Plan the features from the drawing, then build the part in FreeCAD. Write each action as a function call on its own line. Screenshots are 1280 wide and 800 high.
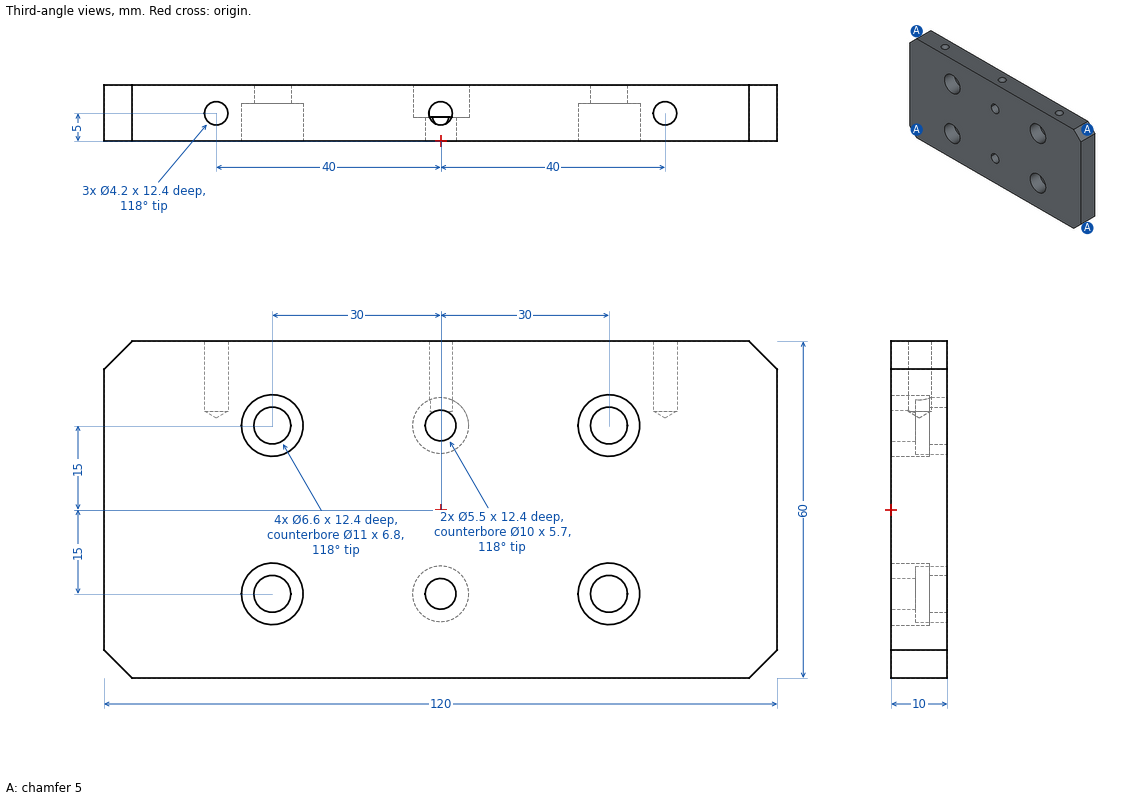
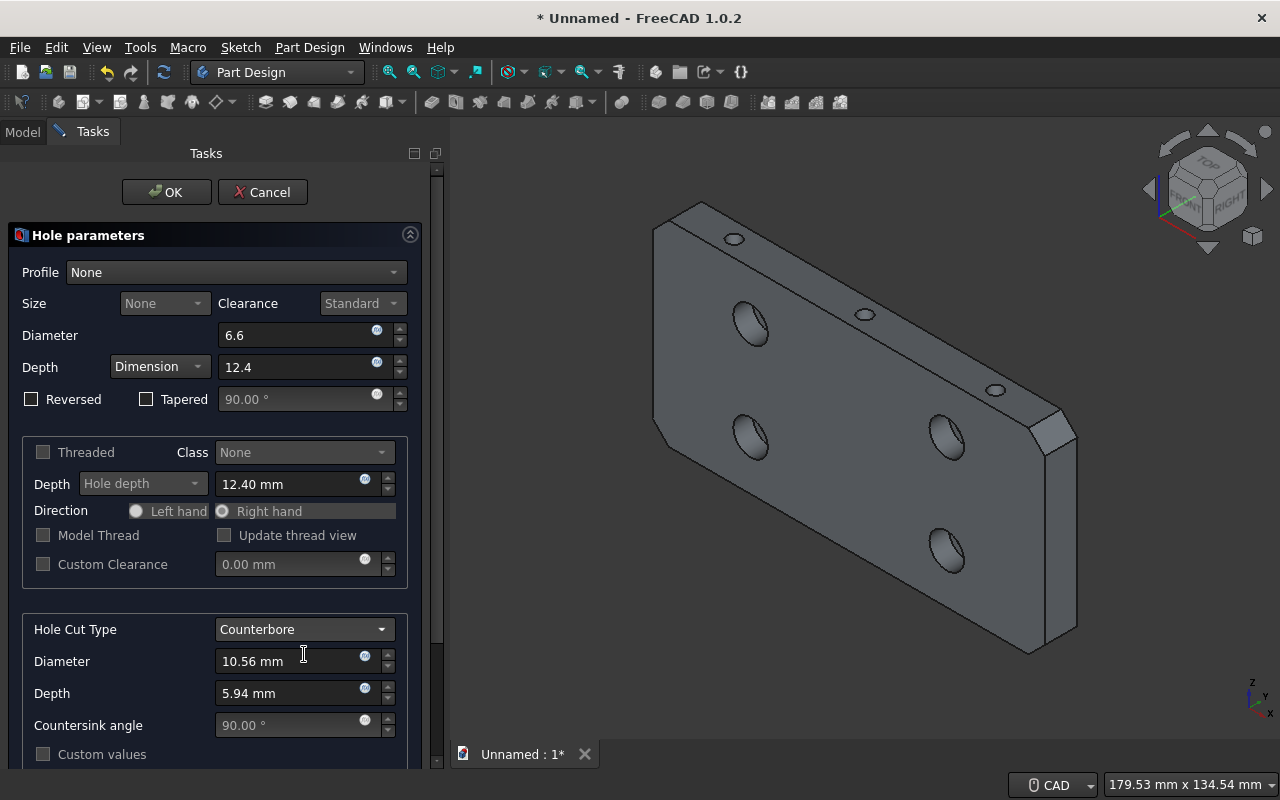
triple_click(298, 661)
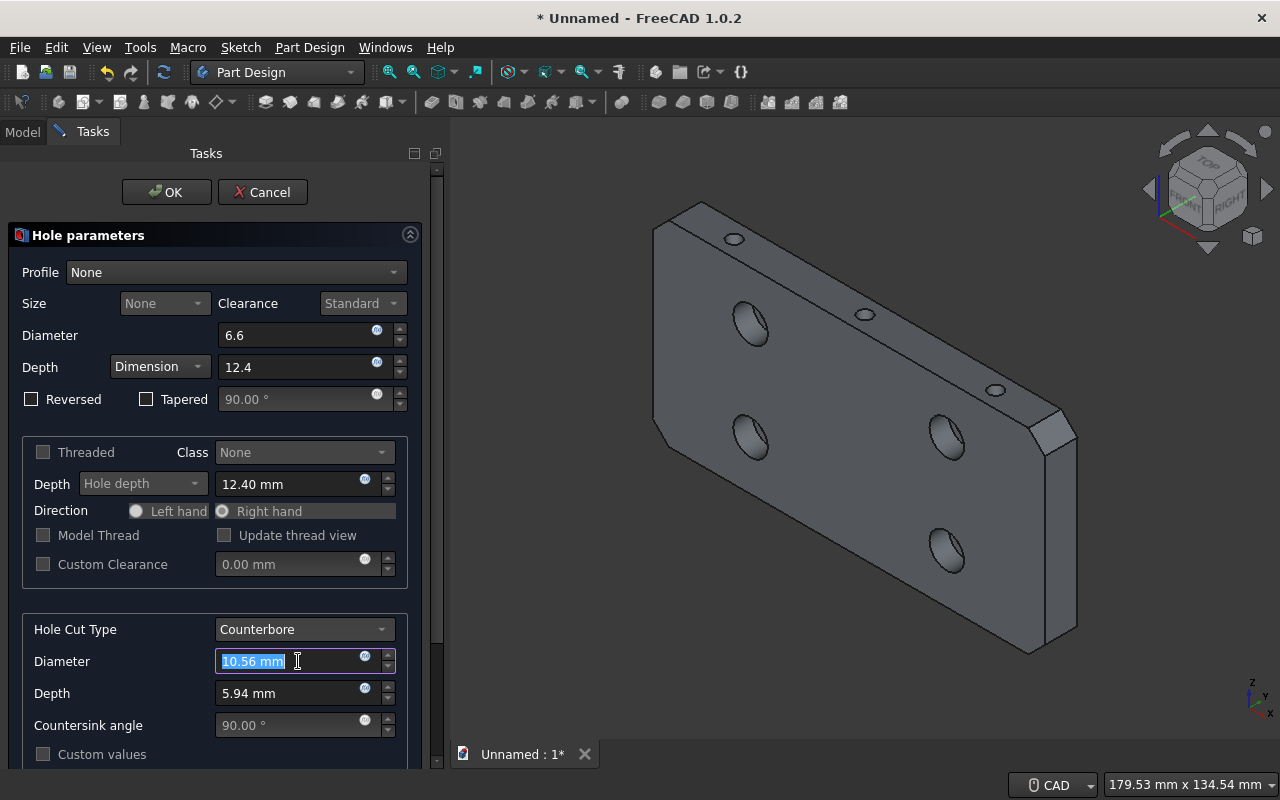
text(11)
key(Tab)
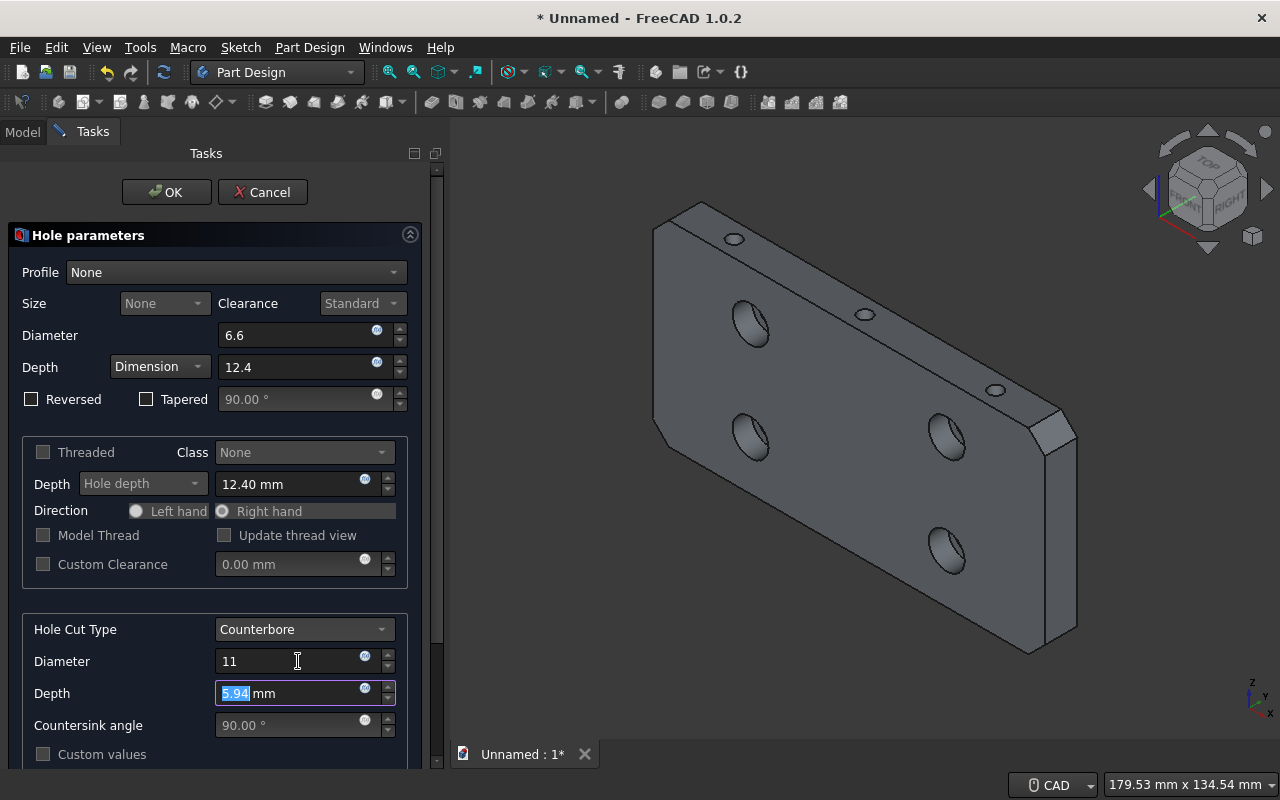
text(6.8)
key(Tab)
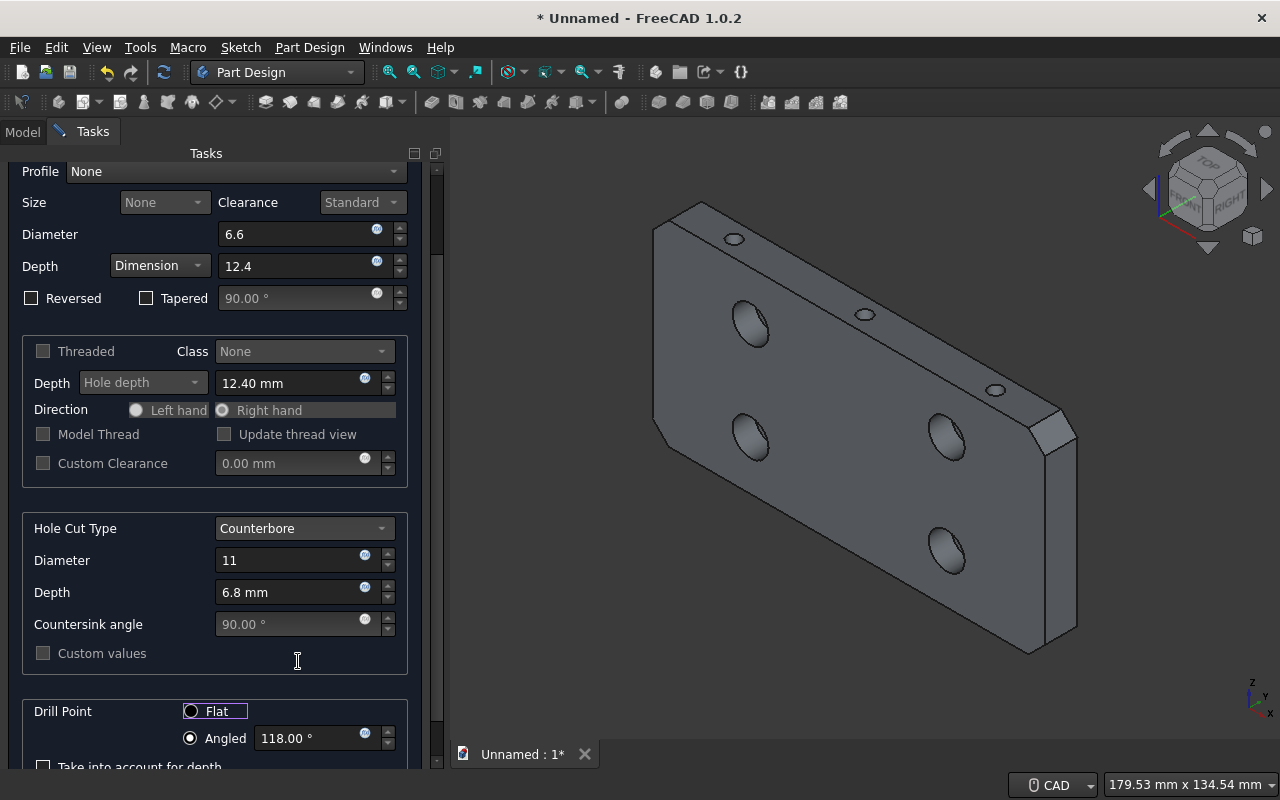
scroll(437, 466, up, 3)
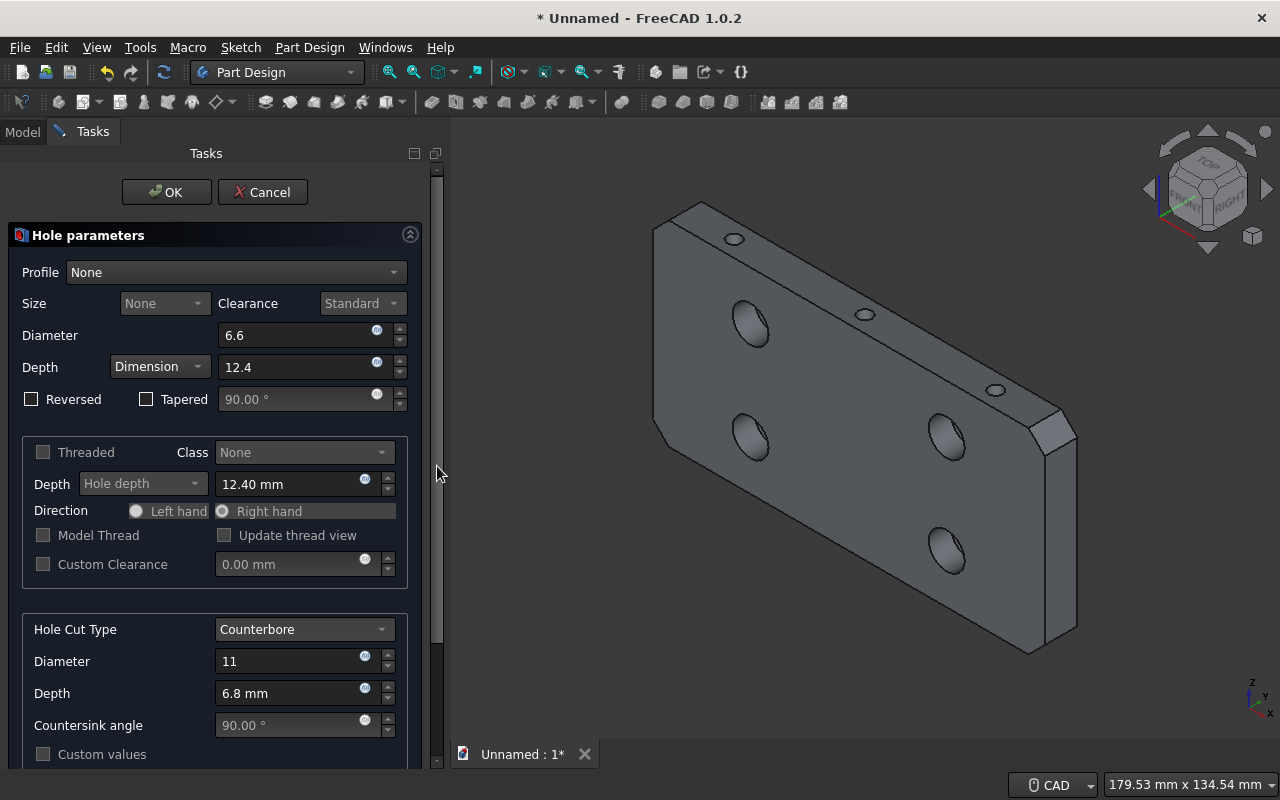
click(167, 192)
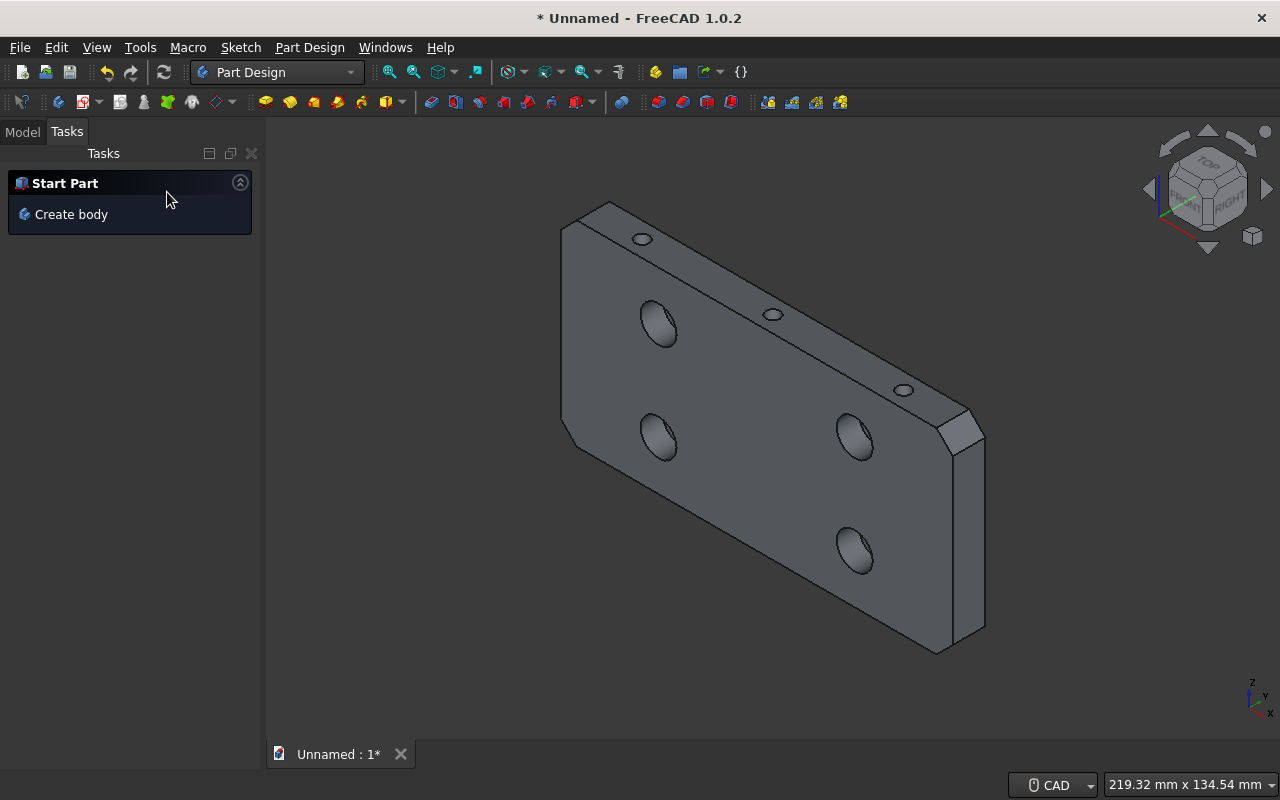
key(4)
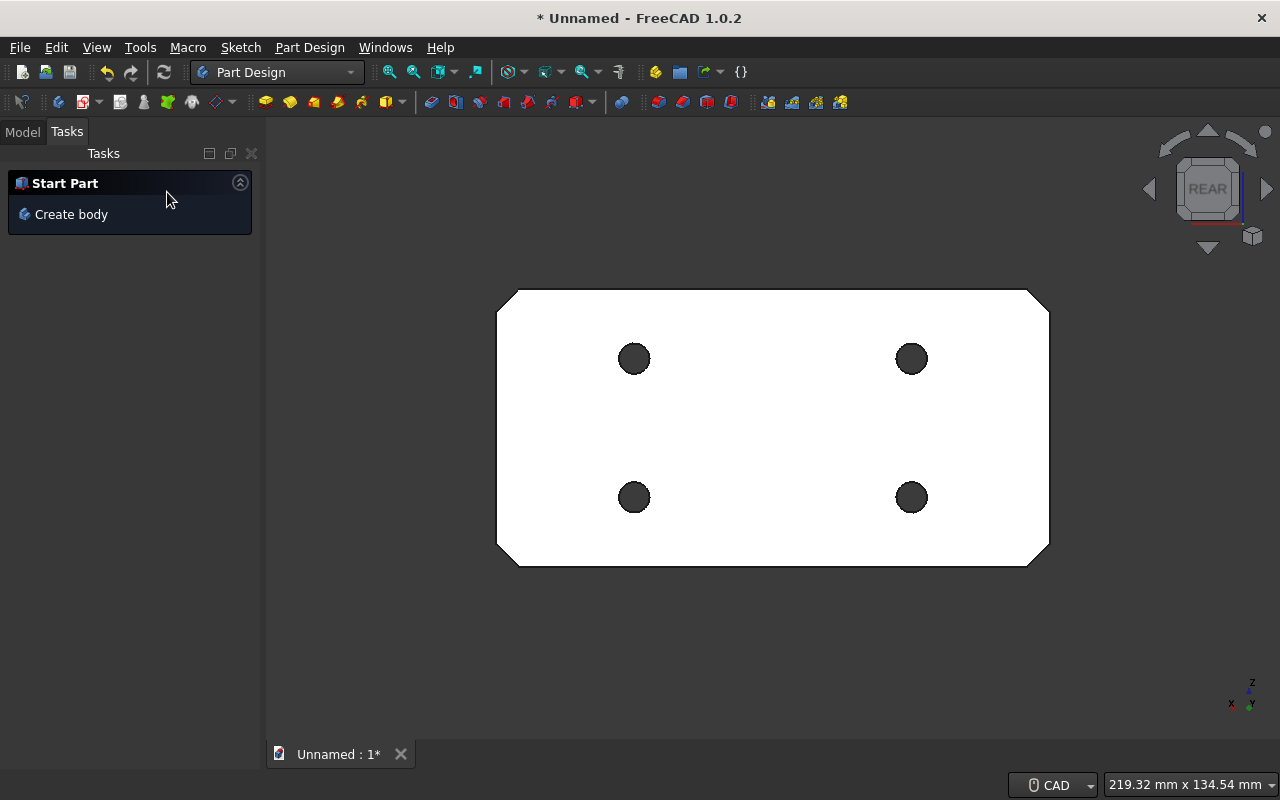
click(773, 427)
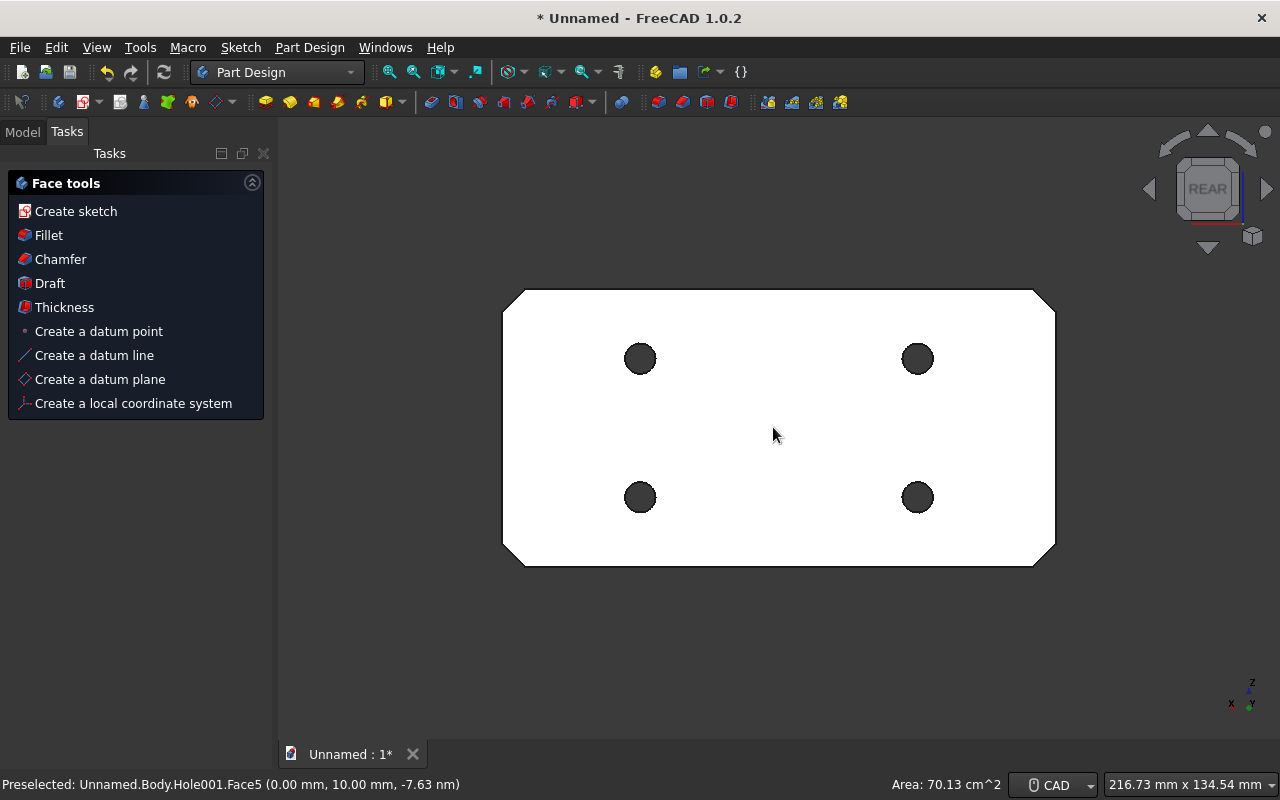
click(84, 102)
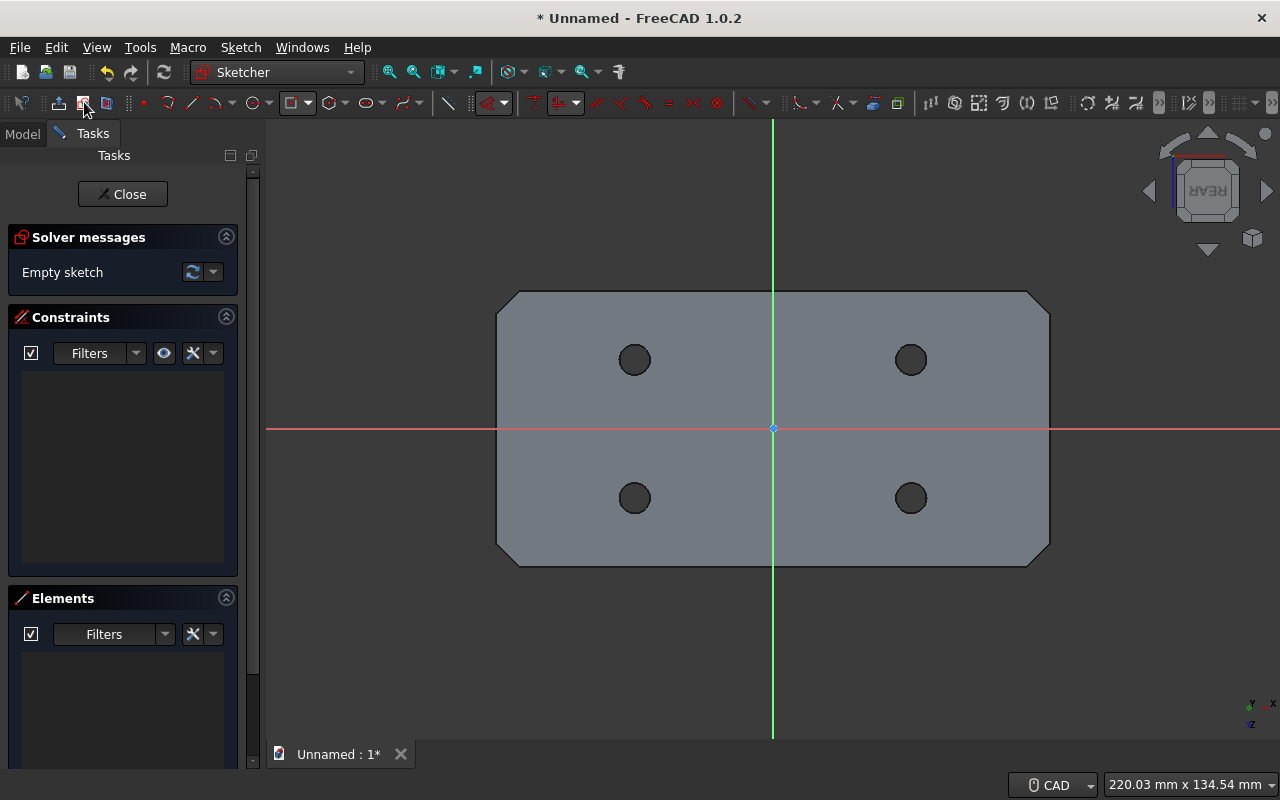
scroll(829, 429, up, 4)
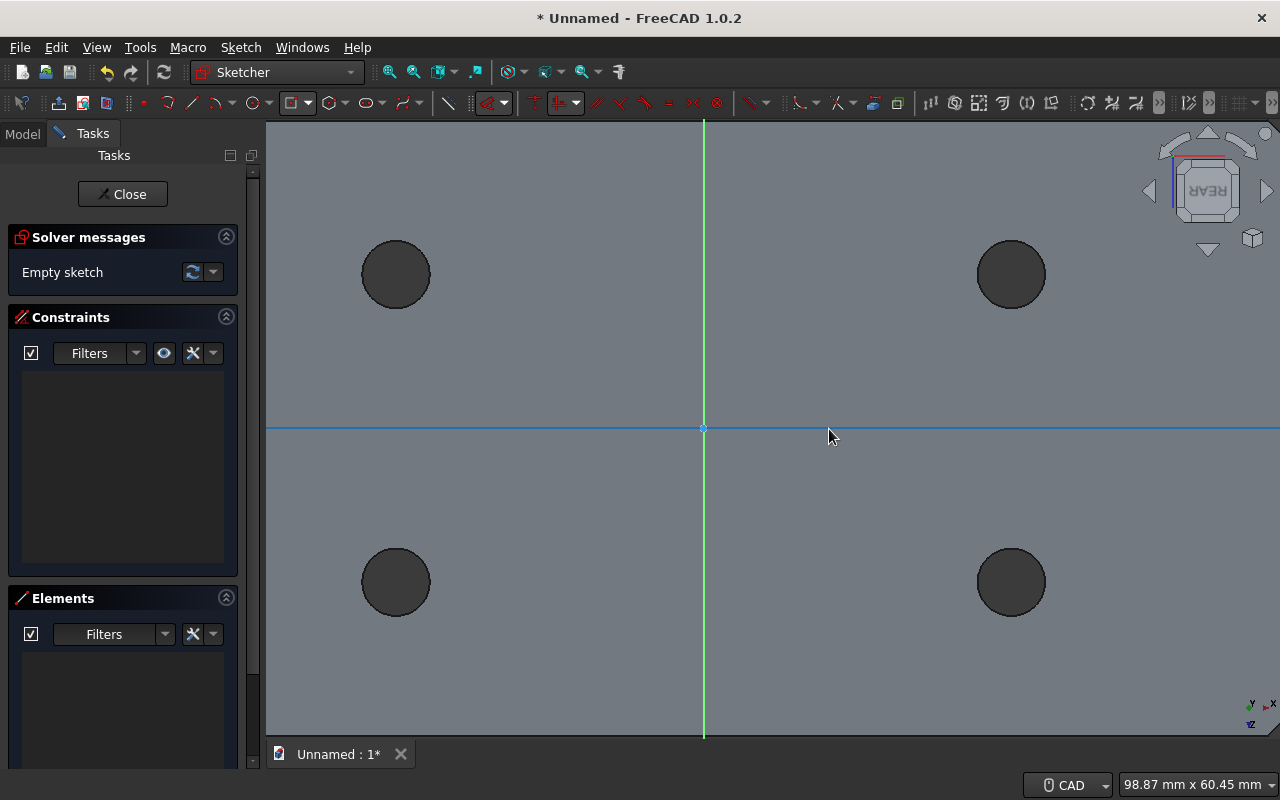
key(g)
key(c)